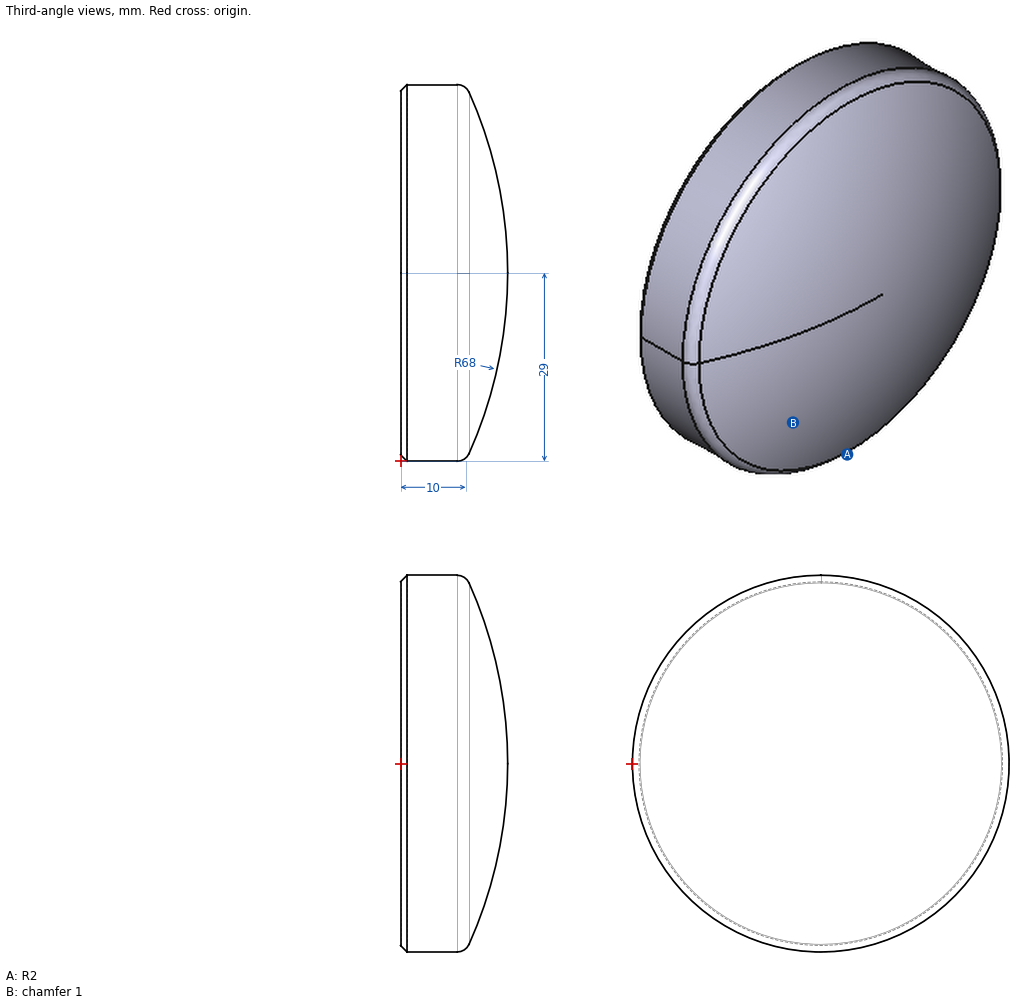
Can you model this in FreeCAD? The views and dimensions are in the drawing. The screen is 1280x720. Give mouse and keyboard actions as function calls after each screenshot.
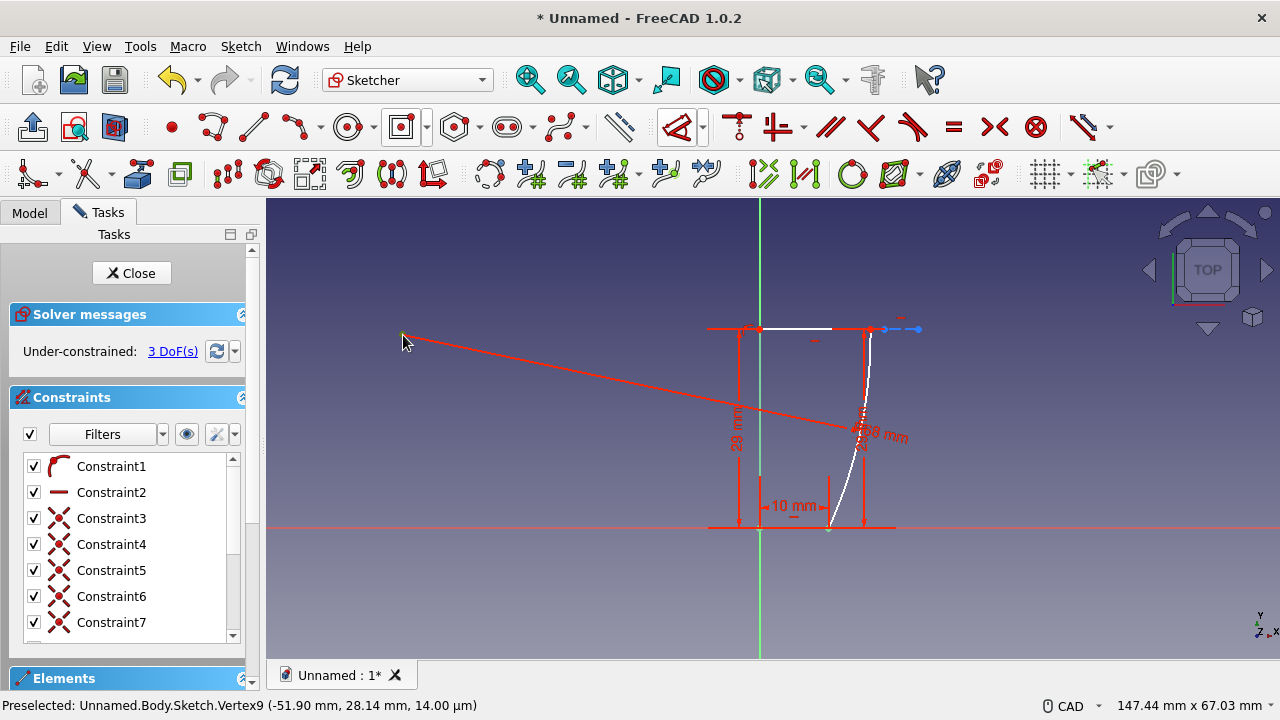
key(i)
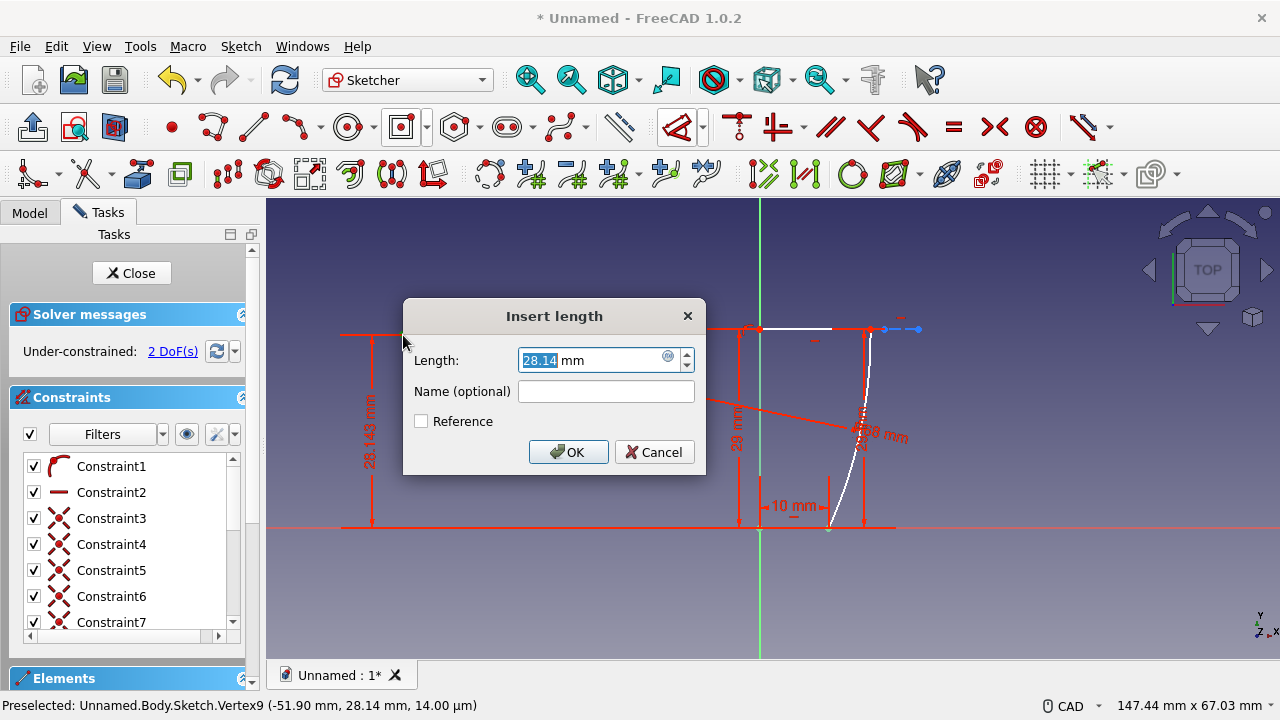
text(29)
key(Return)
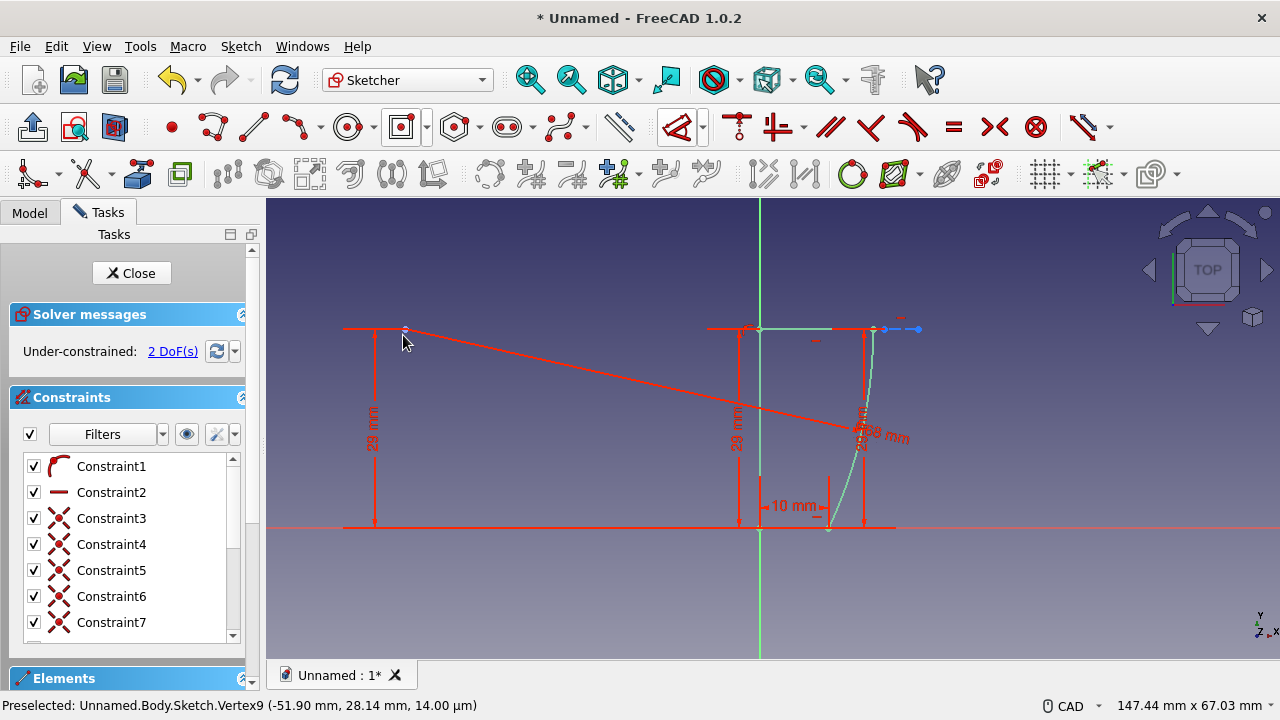
click(132, 273)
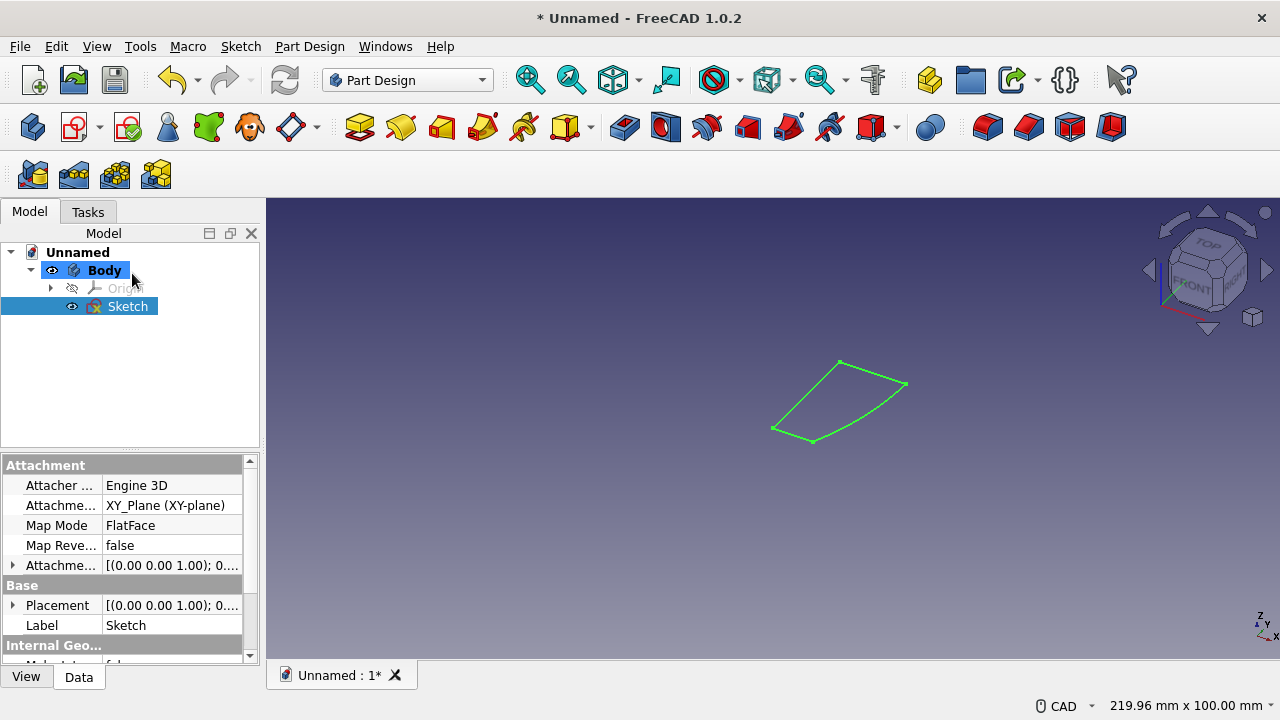
click(401, 128)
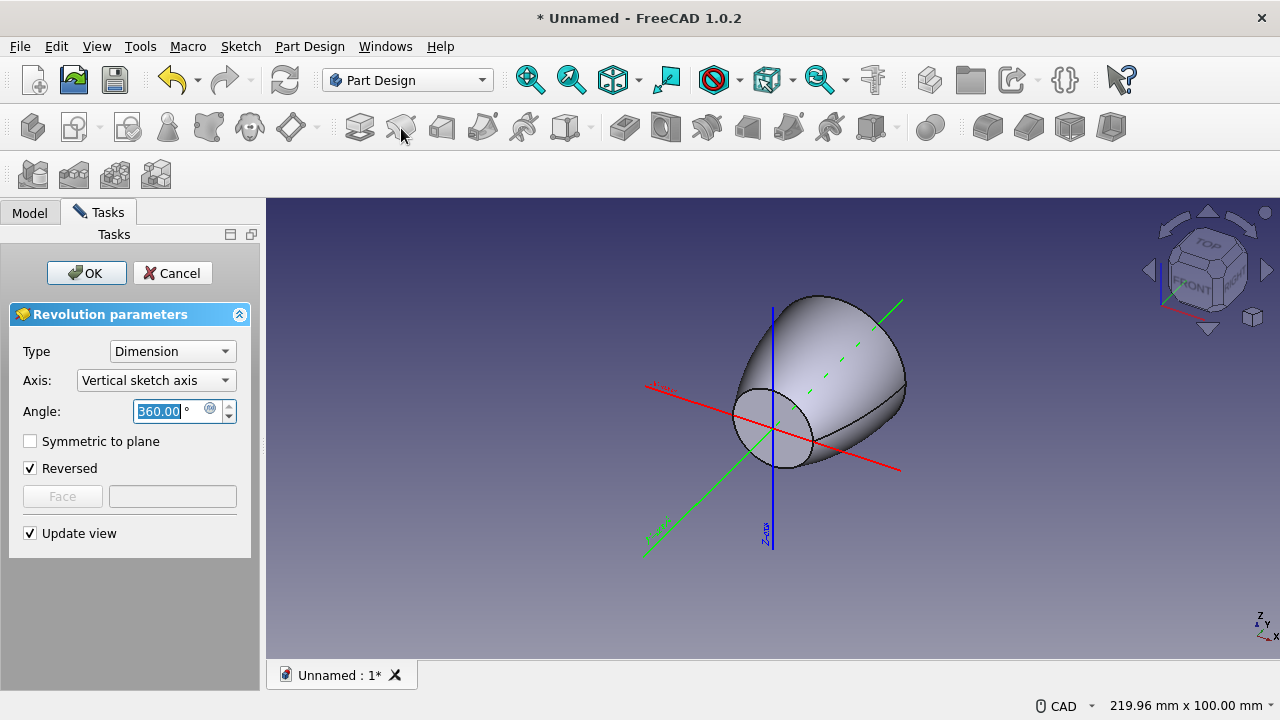
click(157, 380)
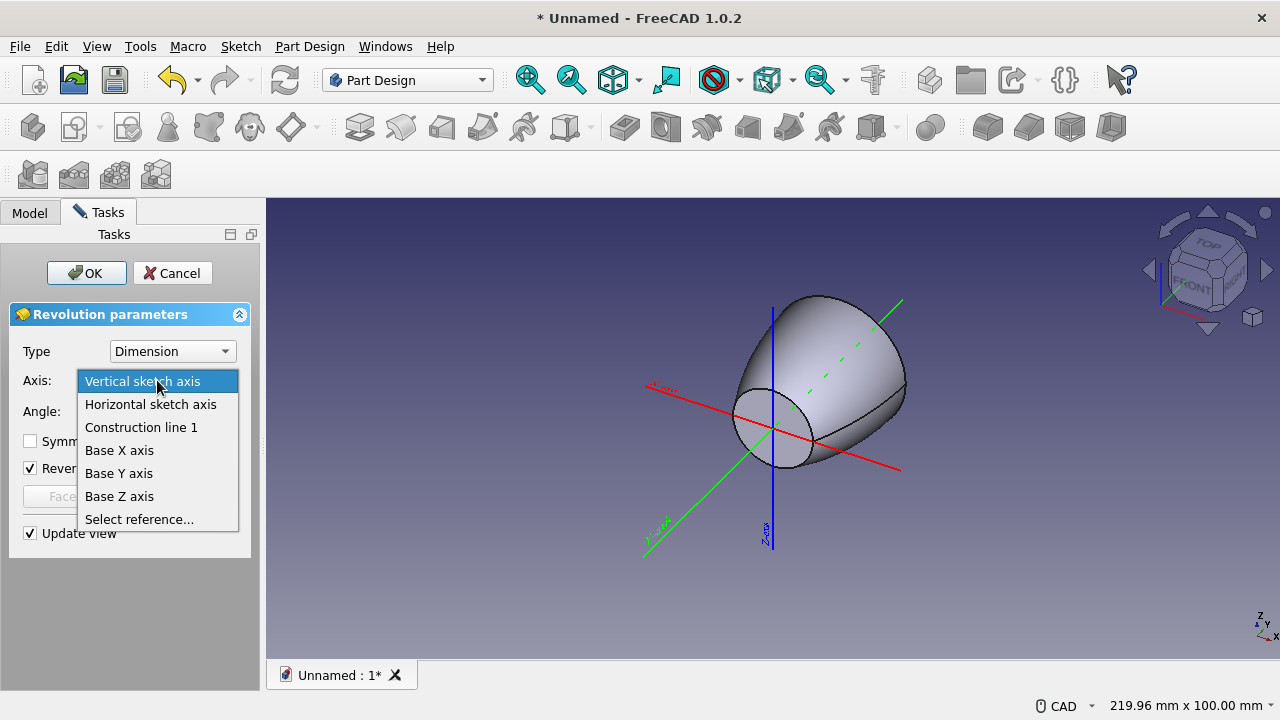
click(156, 428)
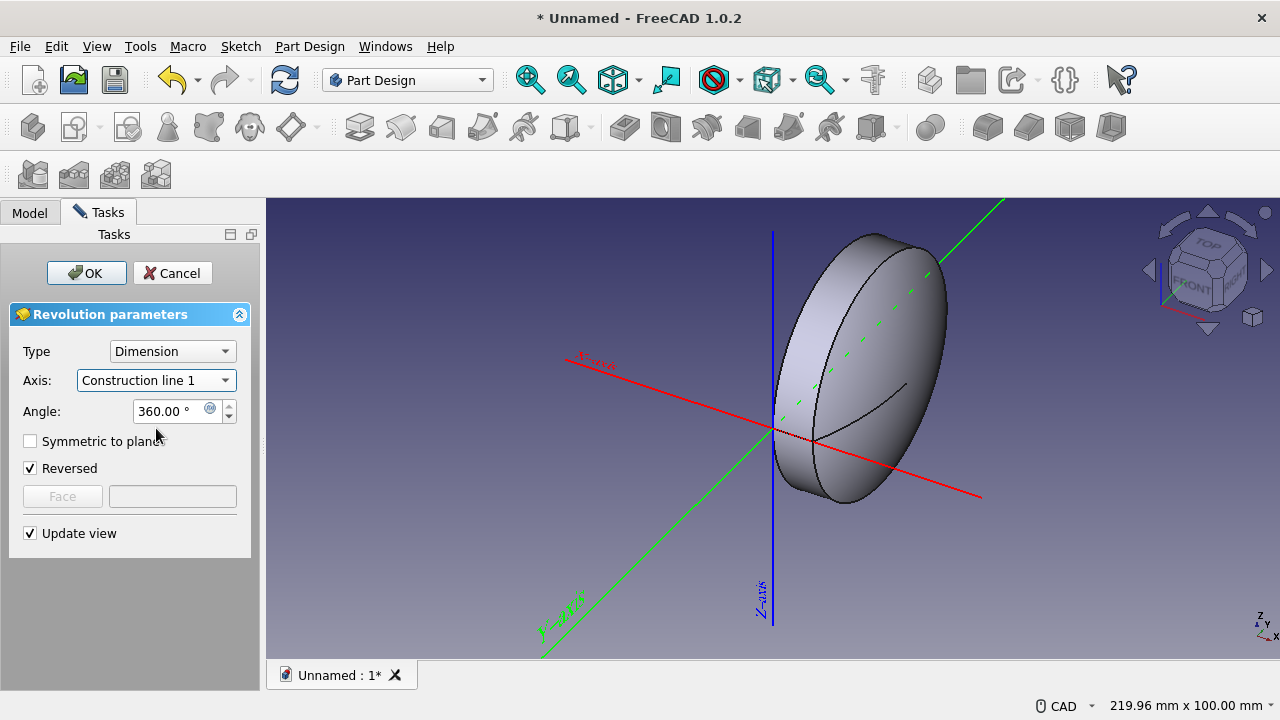
click(87, 273)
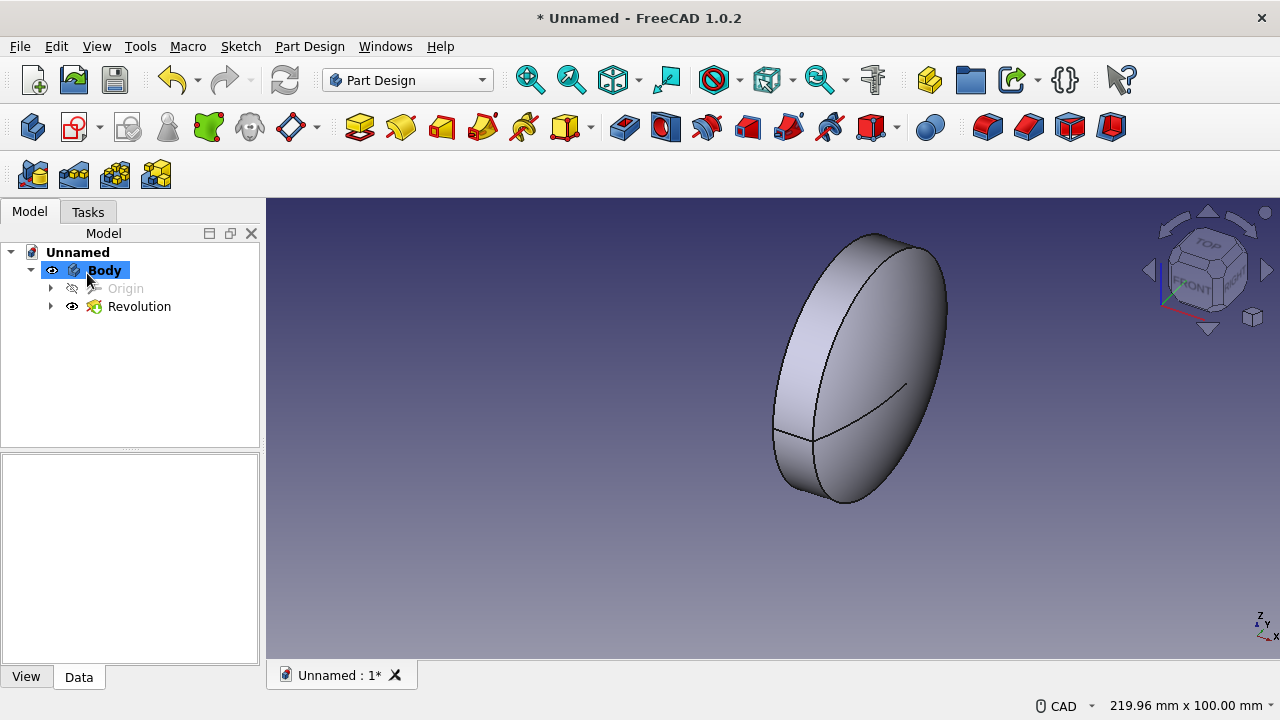
click(531, 80)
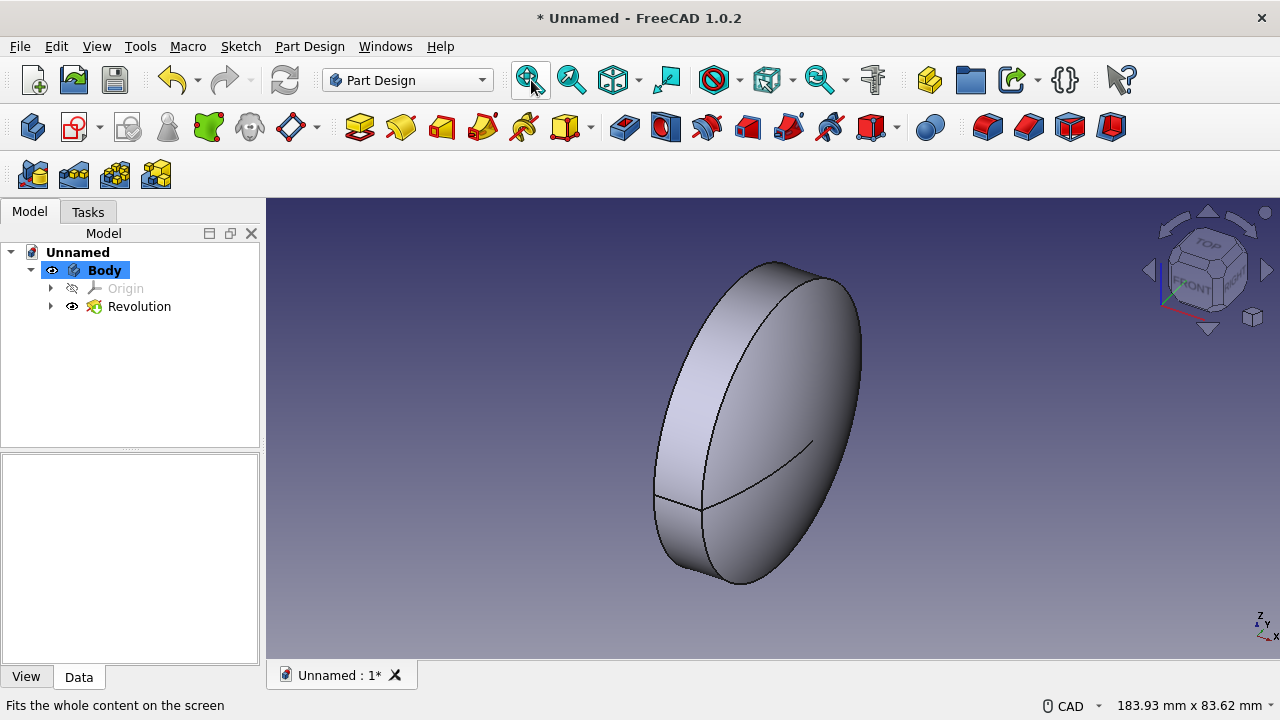
click(806, 281)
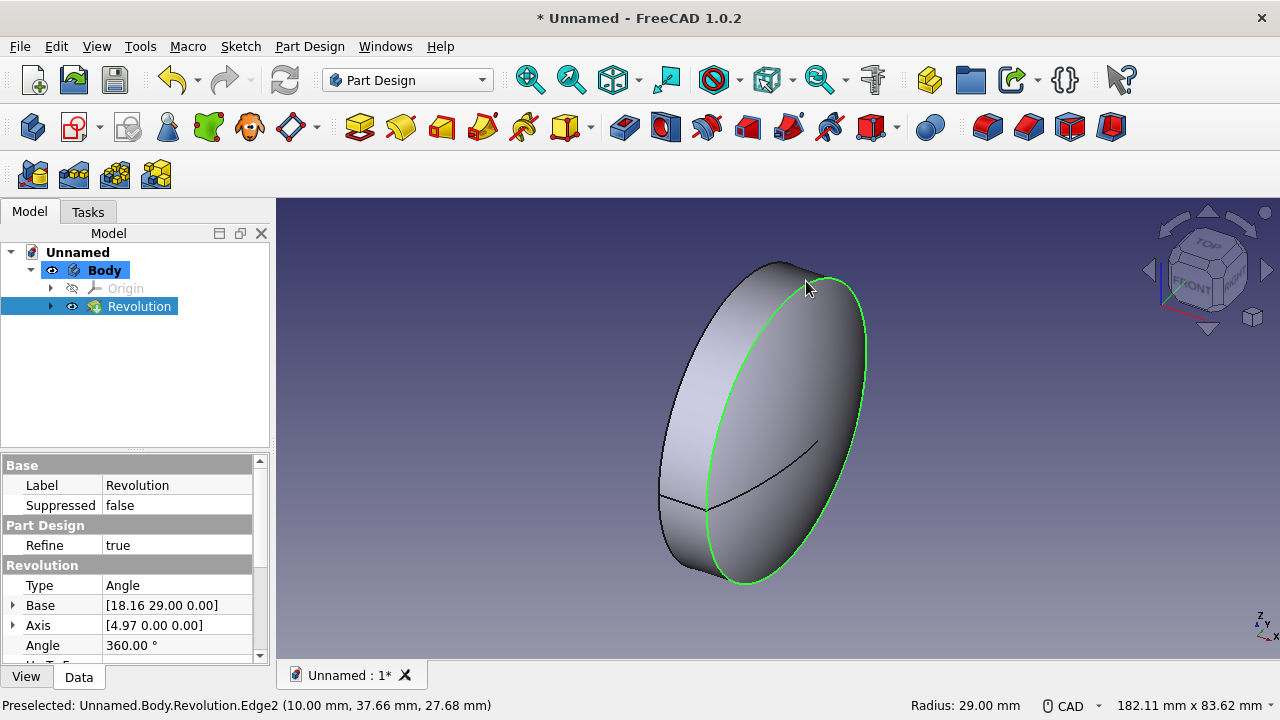
click(988, 128)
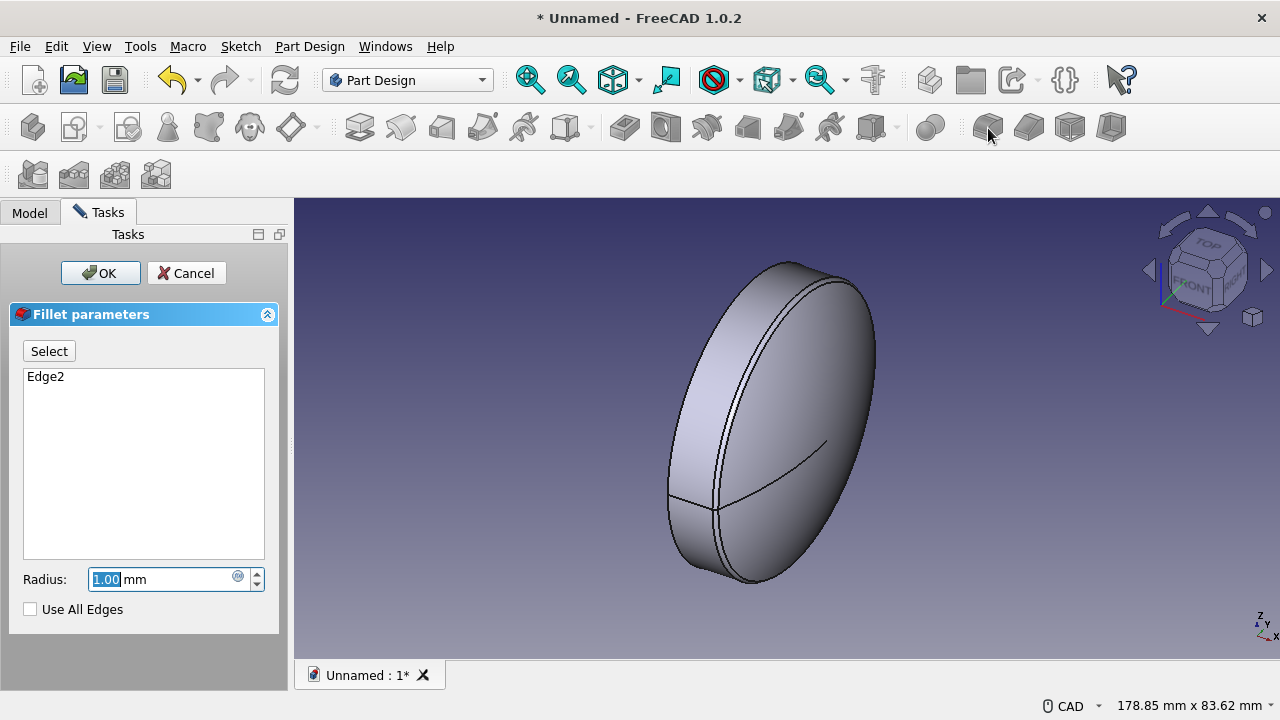
text(2)
key(Tab)